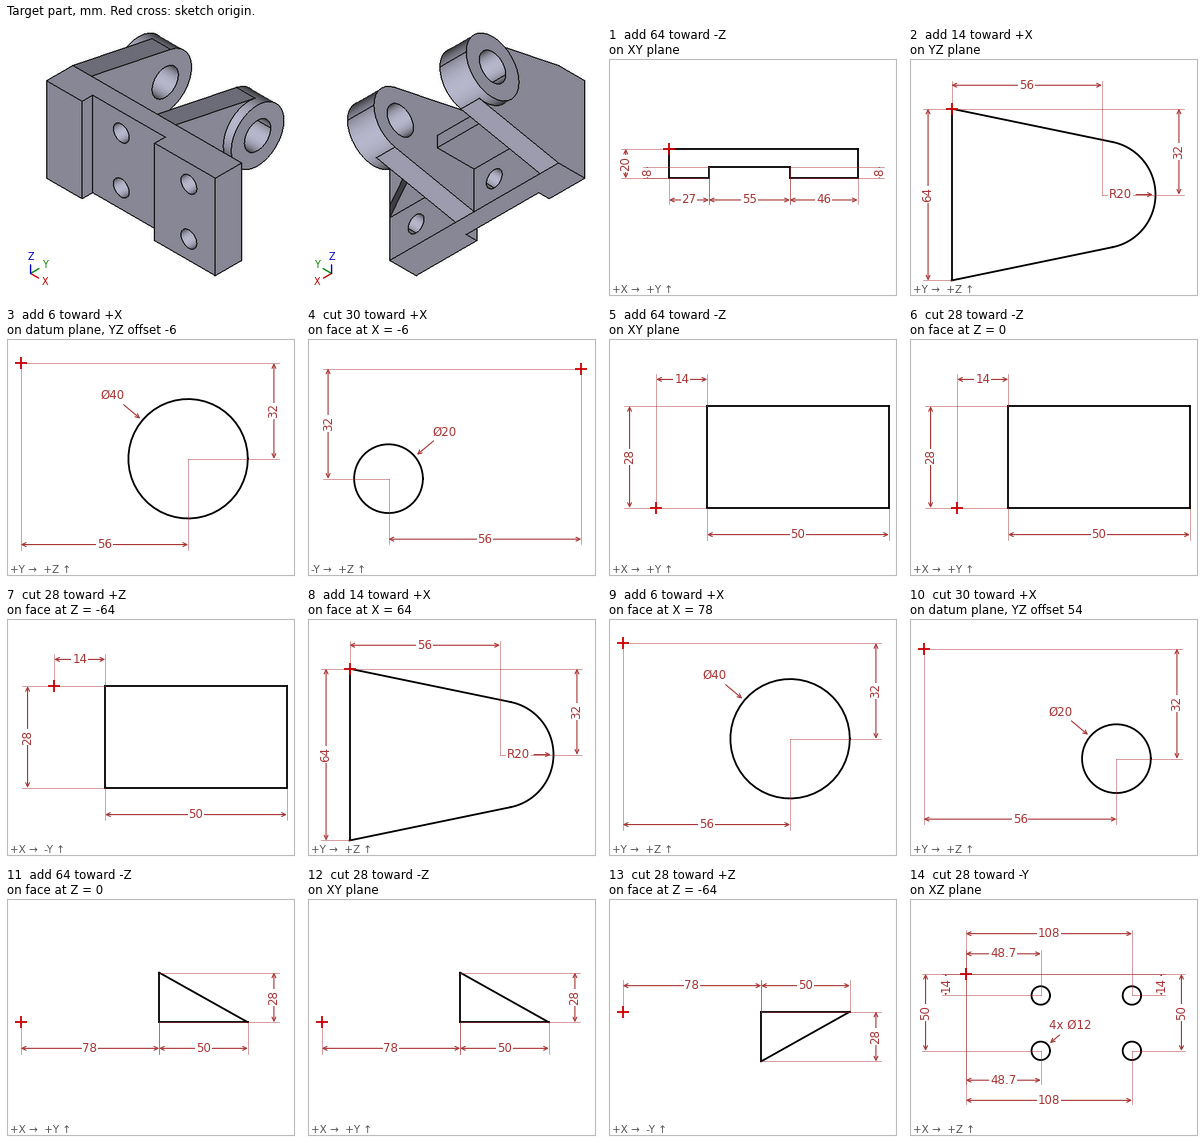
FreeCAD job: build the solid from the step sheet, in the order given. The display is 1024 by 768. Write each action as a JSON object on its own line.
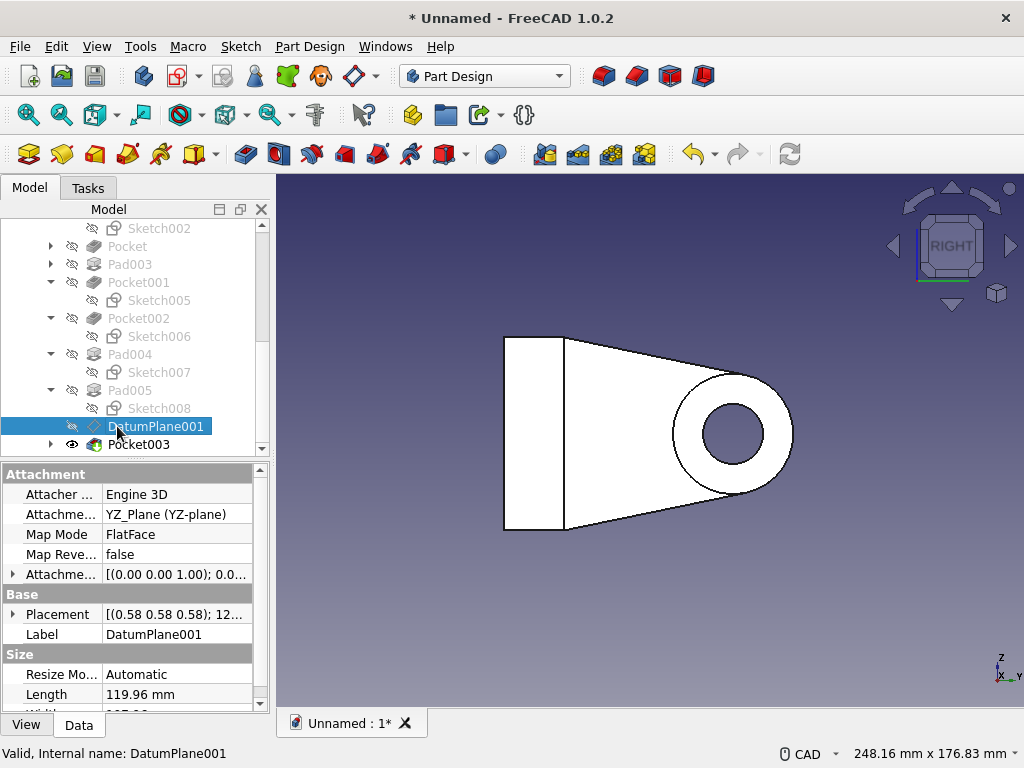
{"action": "left_click", "coordinate": [29, 116]}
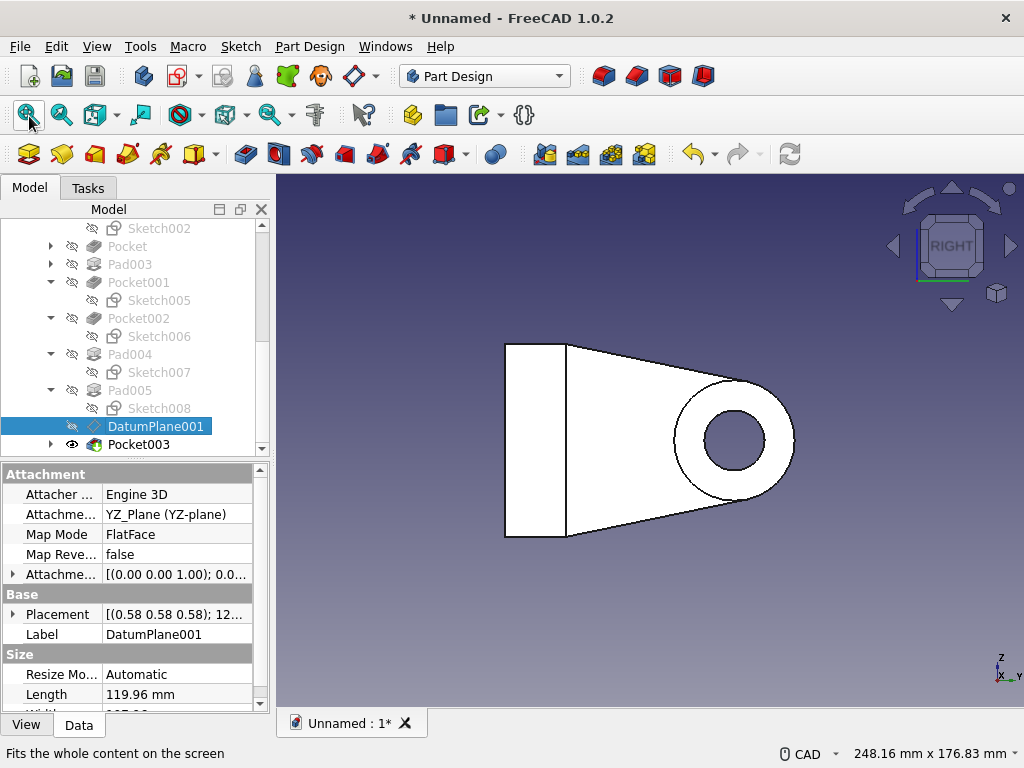
{"action": "key", "text": "0"}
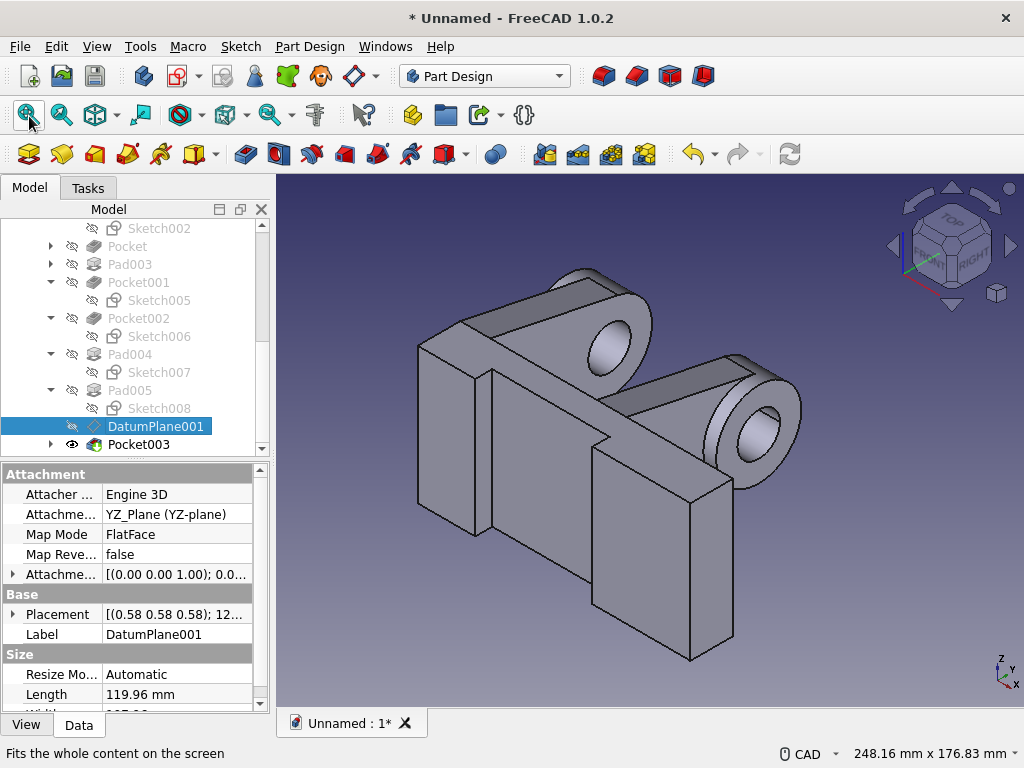
{"action": "left_click", "coordinate": [653, 456]}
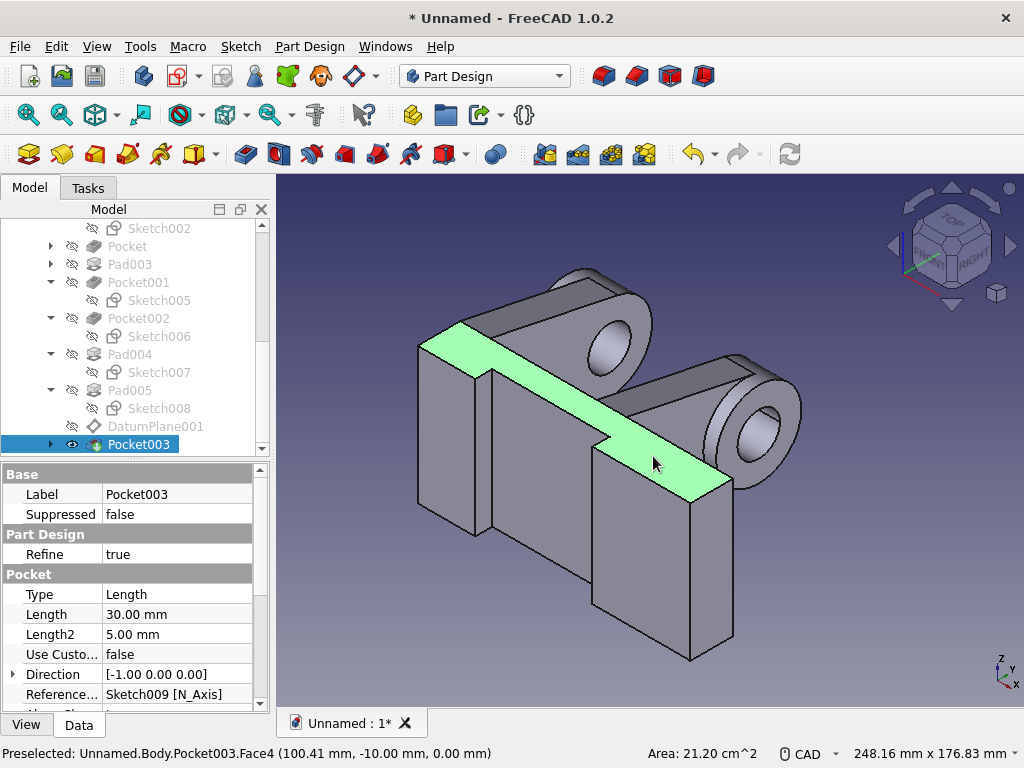
{"action": "left_click", "coordinate": [176, 76]}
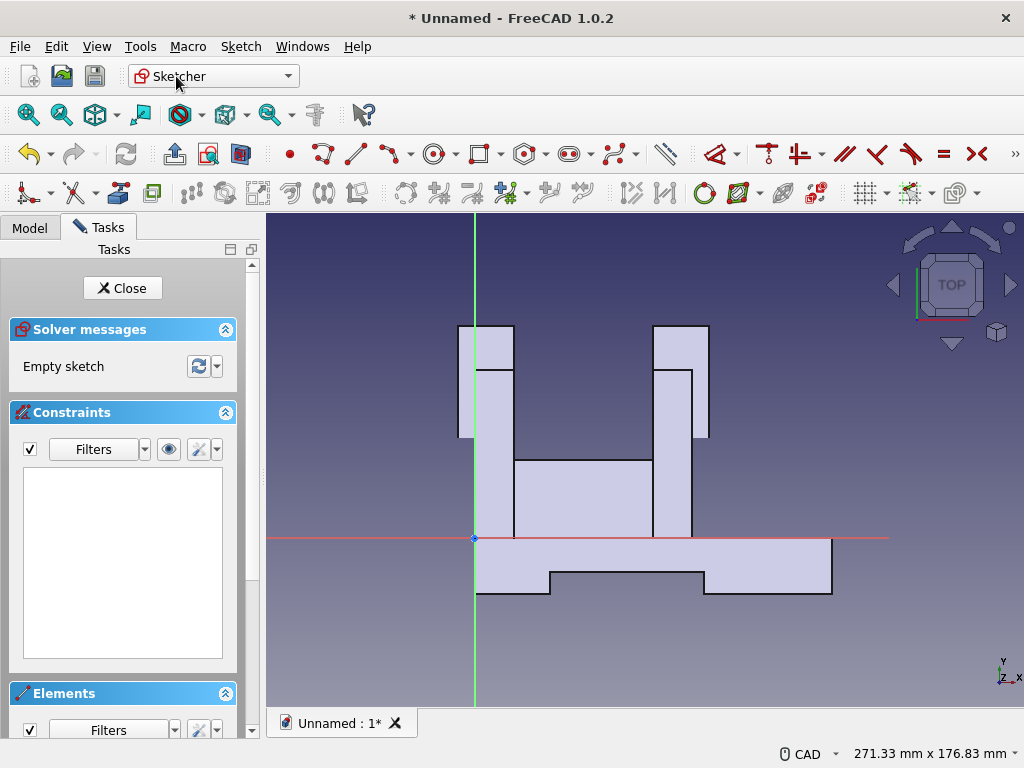
{"action": "scroll", "coordinate": [859, 522], "scroll_direction": "up", "scroll_amount": 5}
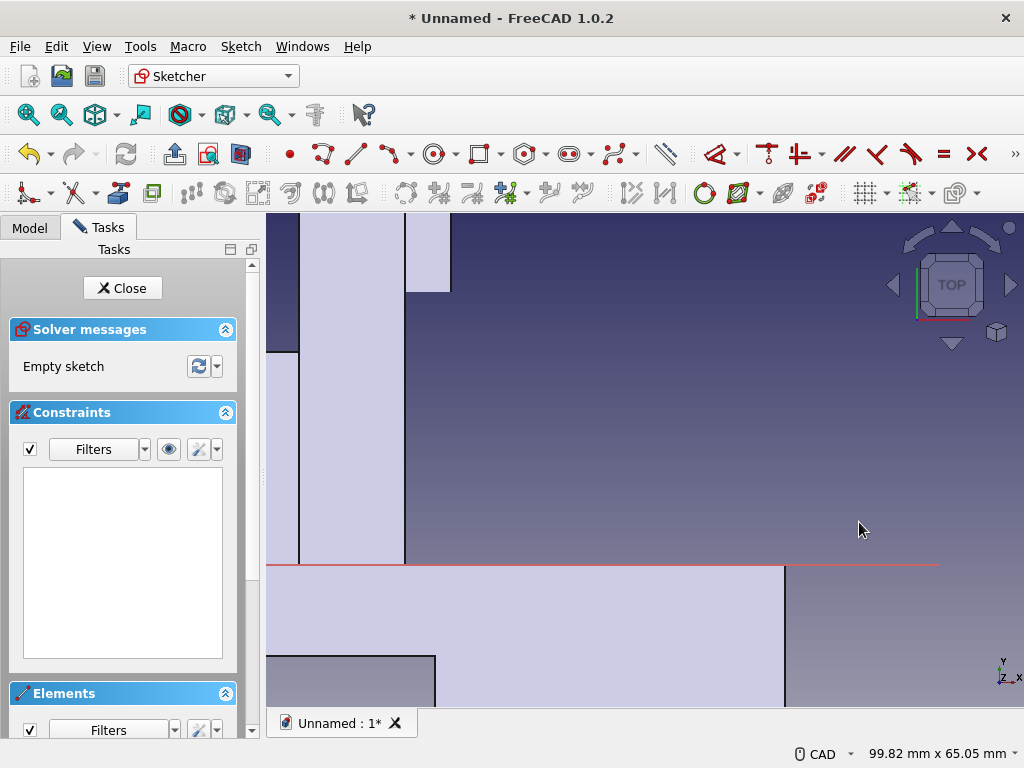
{"action": "left_click", "coordinate": [323, 154]}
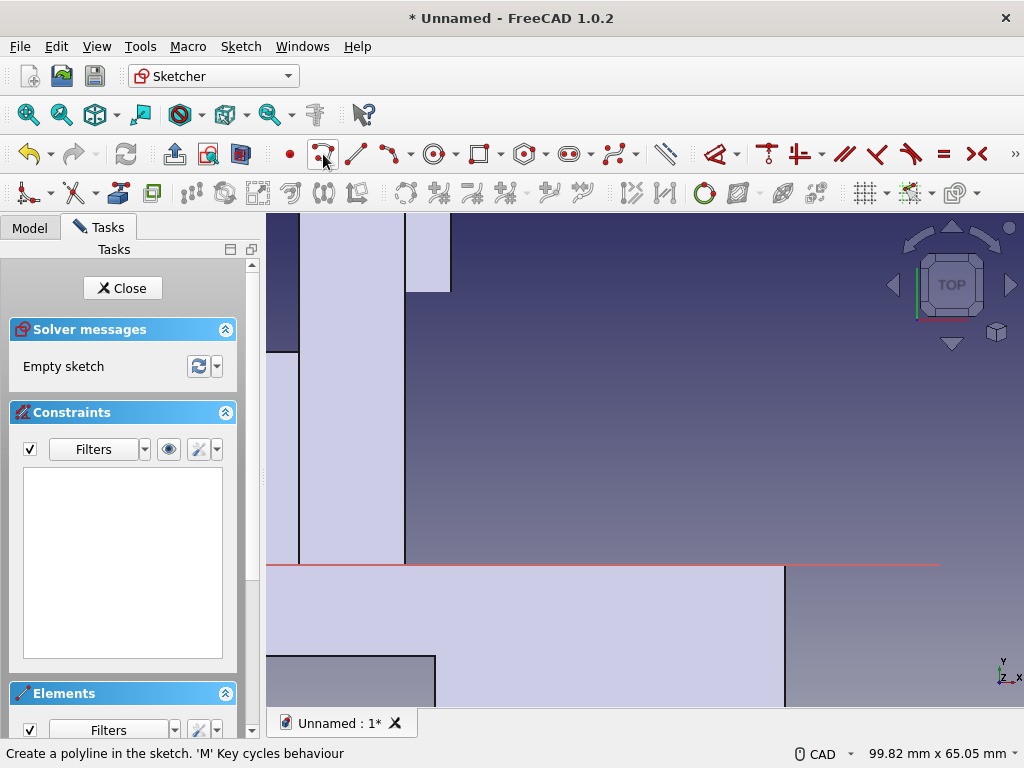
{"action": "left_click", "coordinate": [405, 565]}
{"action": "left_click", "coordinate": [785, 556]}
{"action": "left_click", "coordinate": [405, 352]}
{"action": "left_click", "coordinate": [405, 565]}
{"action": "key", "text": "Escape"}
{"action": "key", "text": "Escape"}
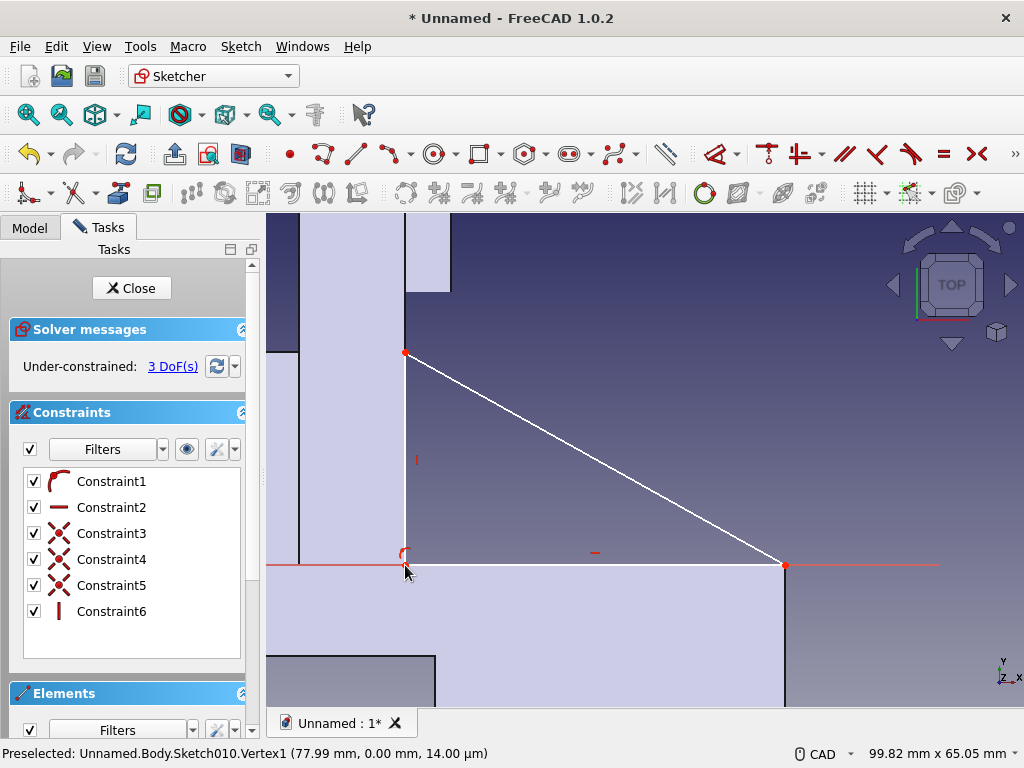
{"action": "left_click", "coordinate": [714, 154]}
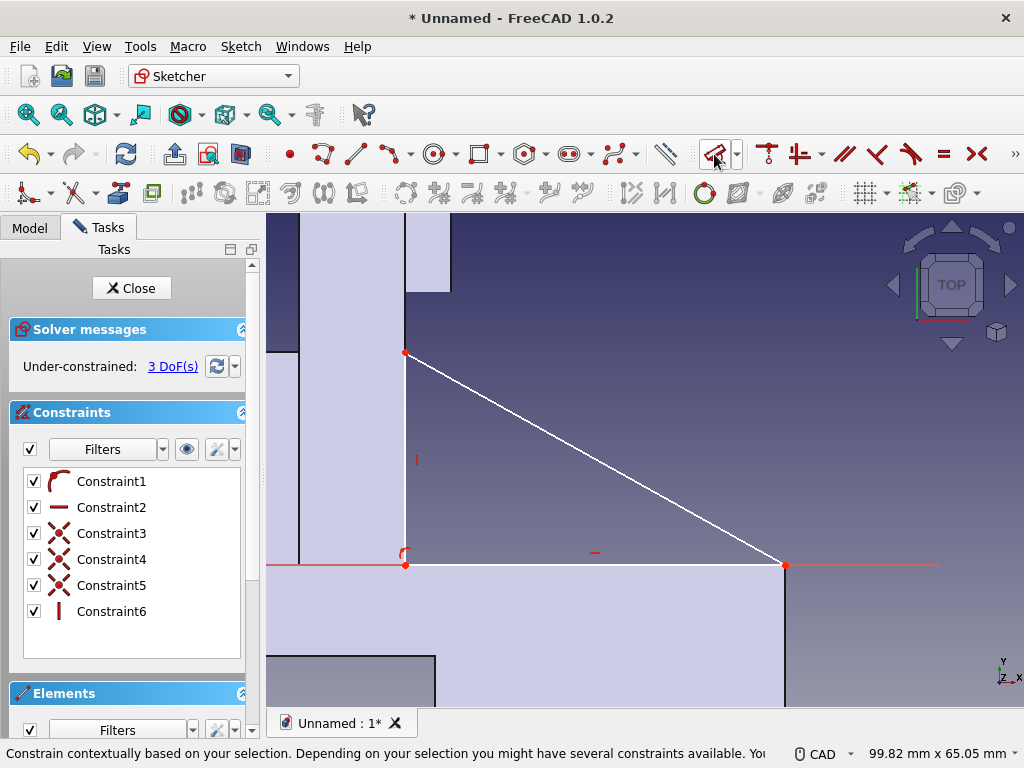
{"action": "left_click", "coordinate": [519, 565]}
{"action": "left_click", "coordinate": [595, 599]}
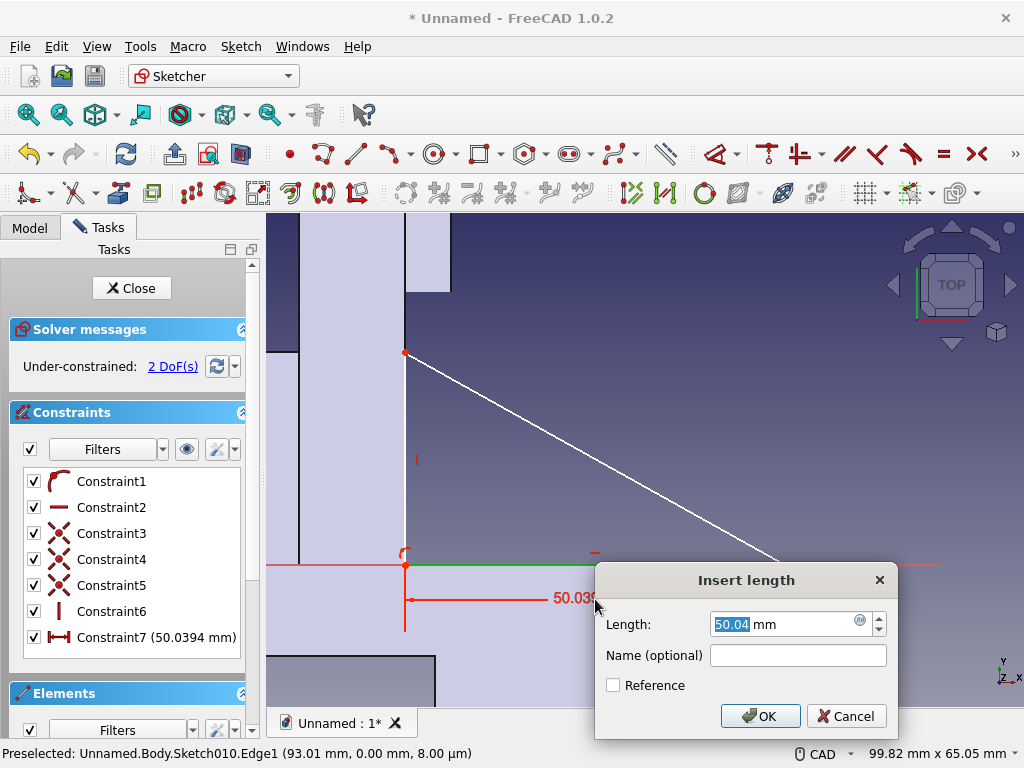
{"action": "type", "text": "50"}
{"action": "key", "text": "Return"}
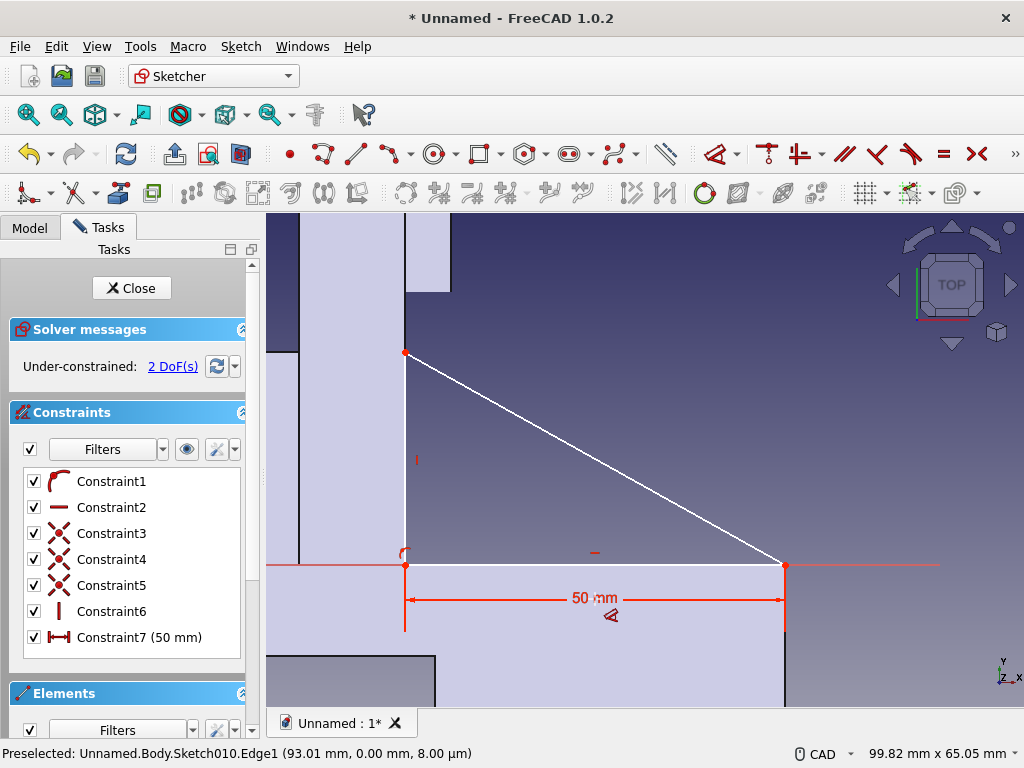
{"action": "left_click", "coordinate": [405, 417]}
{"action": "left_click", "coordinate": [371, 459]}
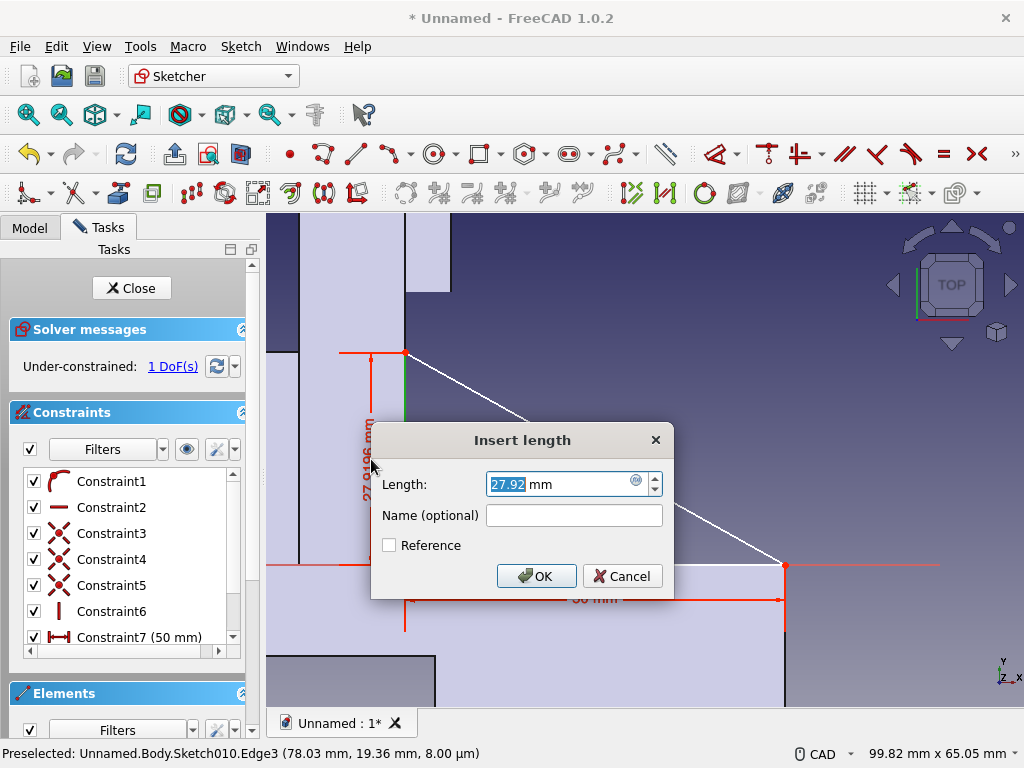
{"action": "type", "text": "28"}
{"action": "key", "text": "Return"}